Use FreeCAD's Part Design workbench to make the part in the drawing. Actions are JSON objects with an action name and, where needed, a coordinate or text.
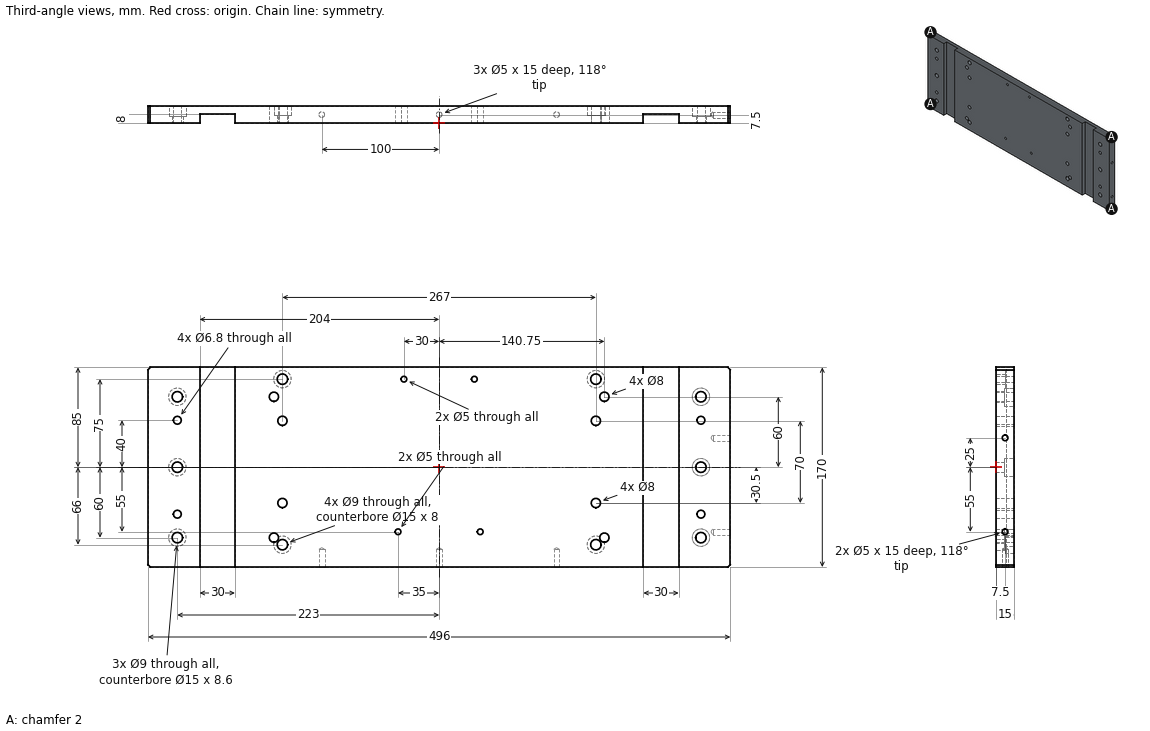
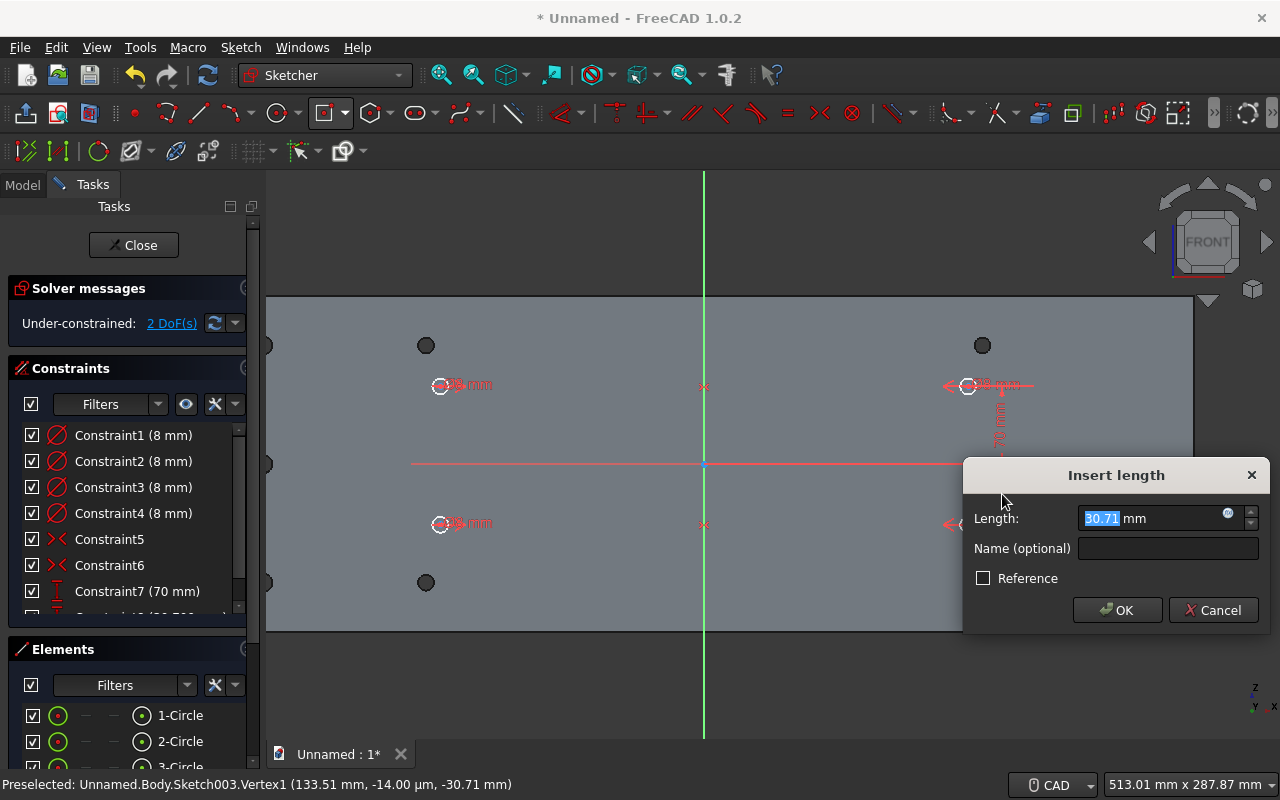
{"action": "type", "text": "30.5"}
{"action": "key", "text": "Return"}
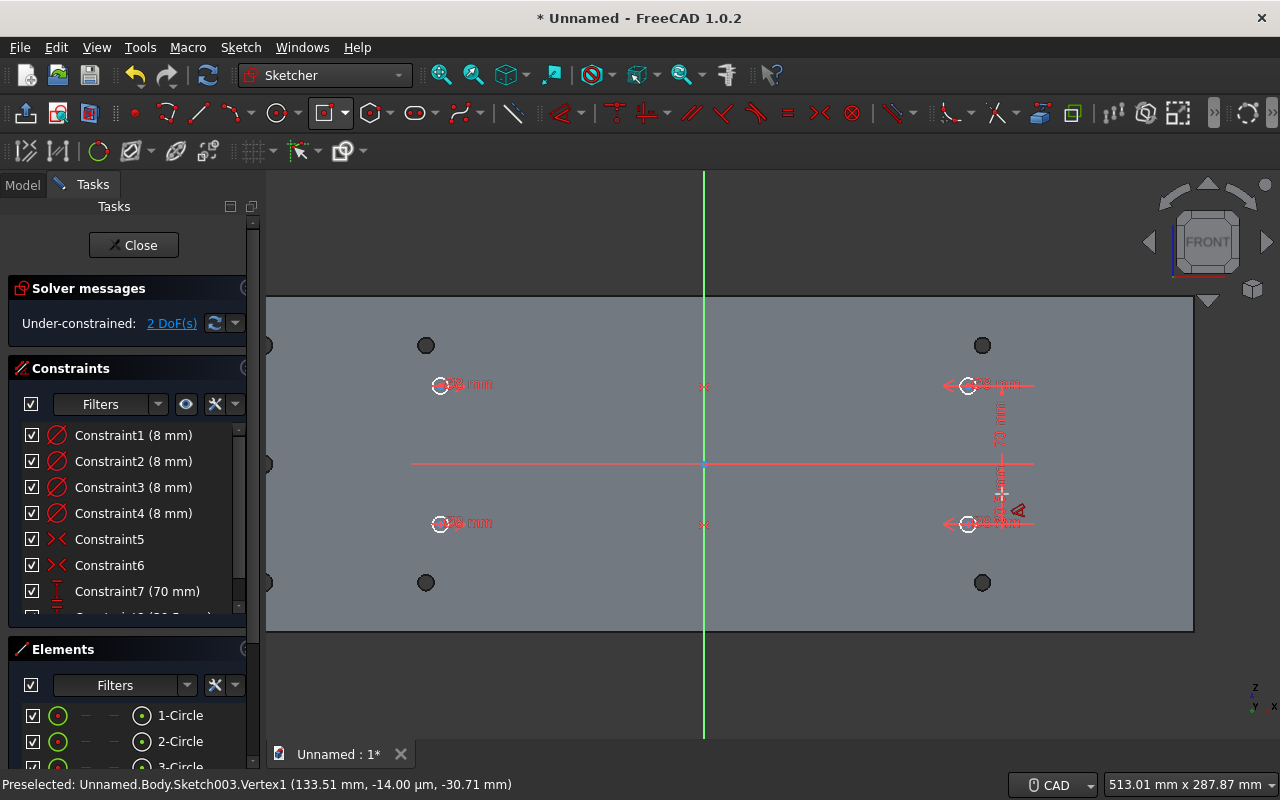
{"action": "left_click", "coordinate": [968, 386]}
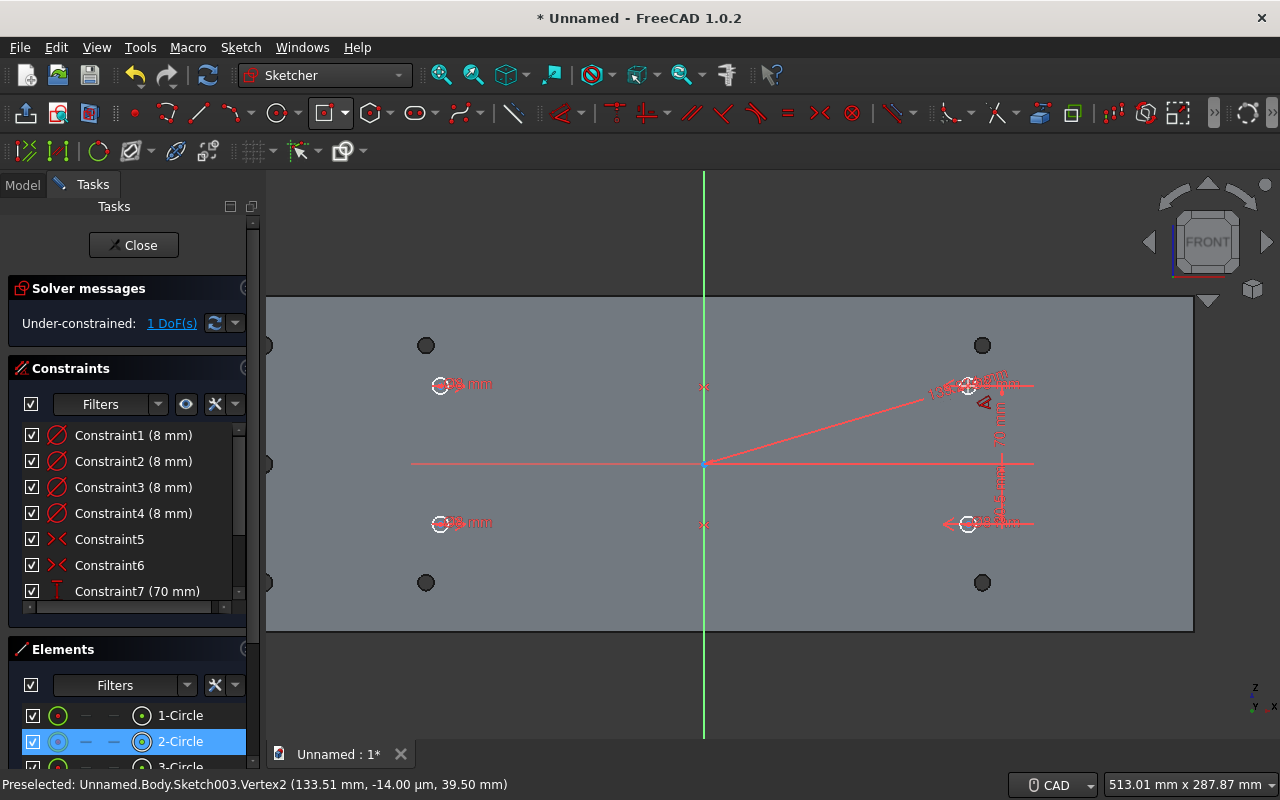
{"action": "left_click", "coordinate": [440, 386]}
{"action": "left_click", "coordinate": [583, 352]}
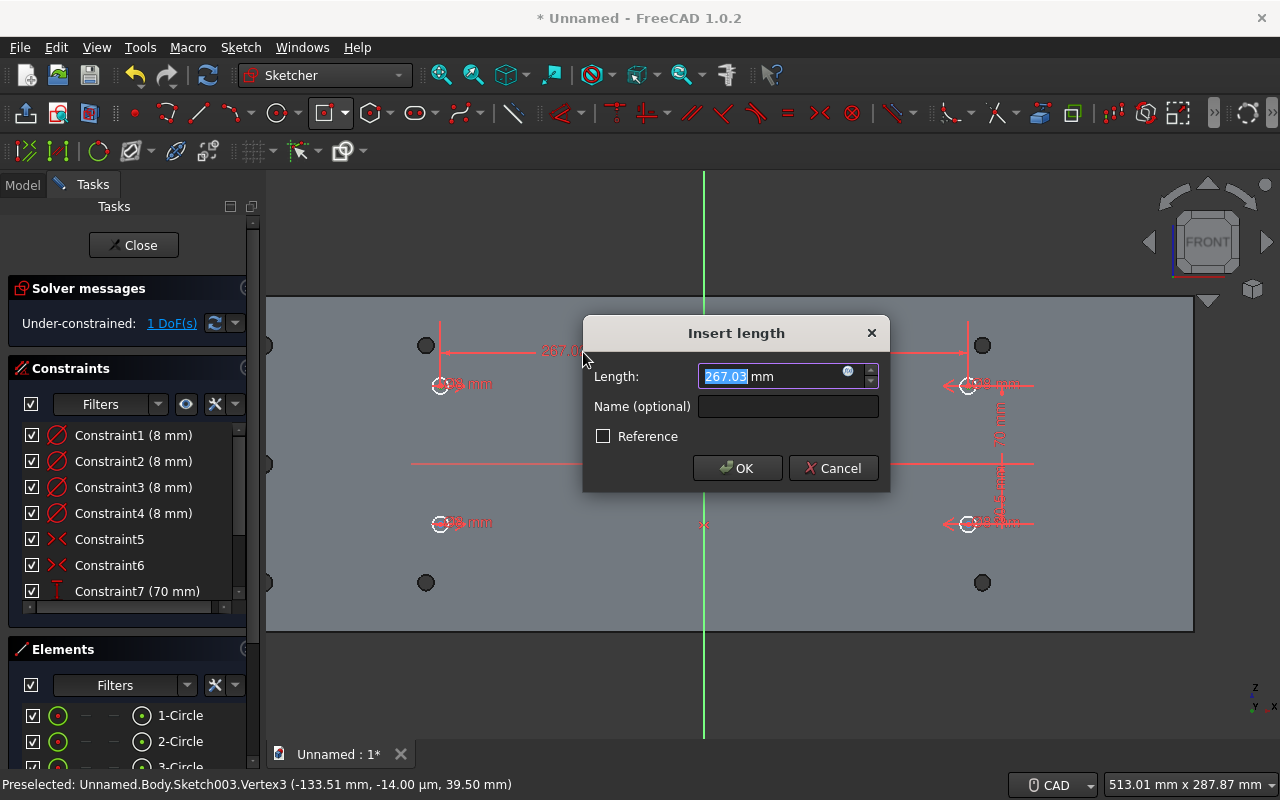
{"action": "type", "text": "267"}
{"action": "key", "text": "Return"}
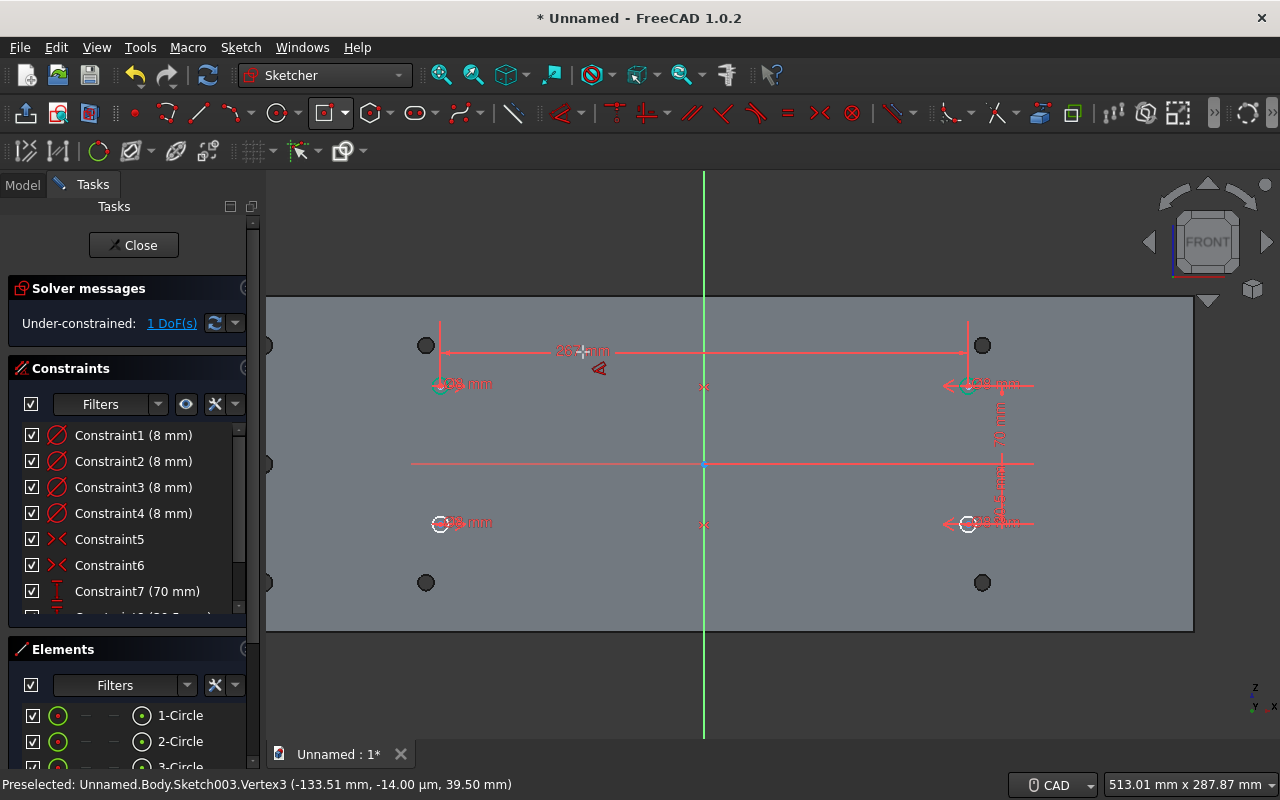
{"action": "left_click", "coordinate": [968, 524]}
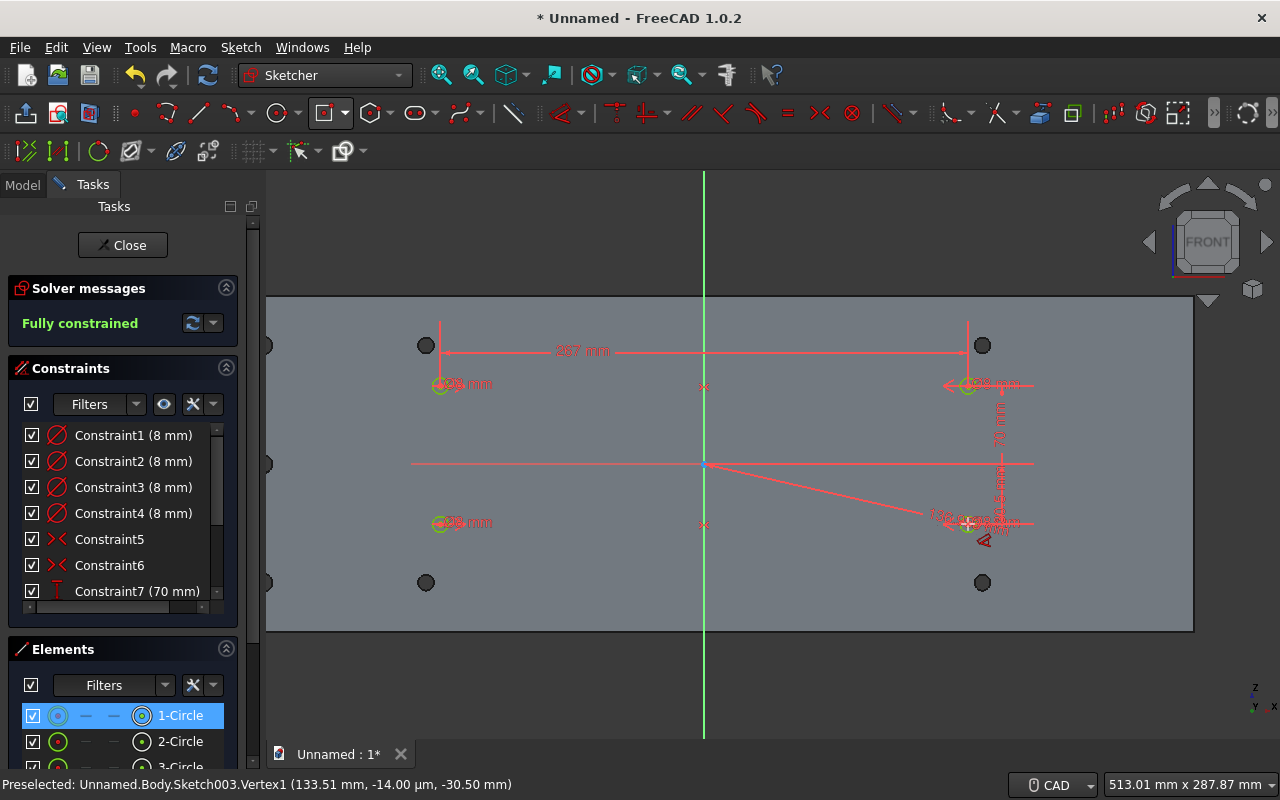
{"action": "left_click", "coordinate": [440, 386]}
{"action": "left_click", "coordinate": [826, 352]}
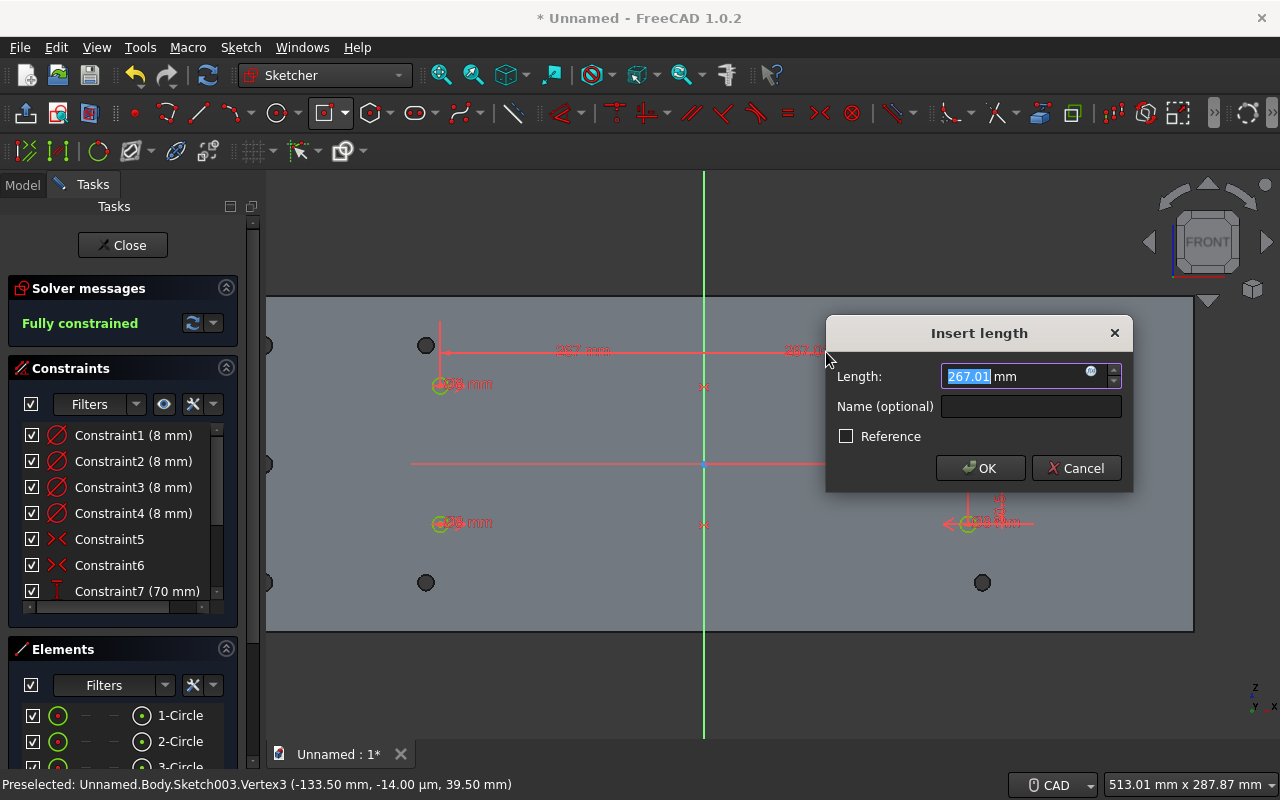
{"action": "type", "text": "267"}
{"action": "key", "text": "Return"}
{"action": "key", "text": "Escape"}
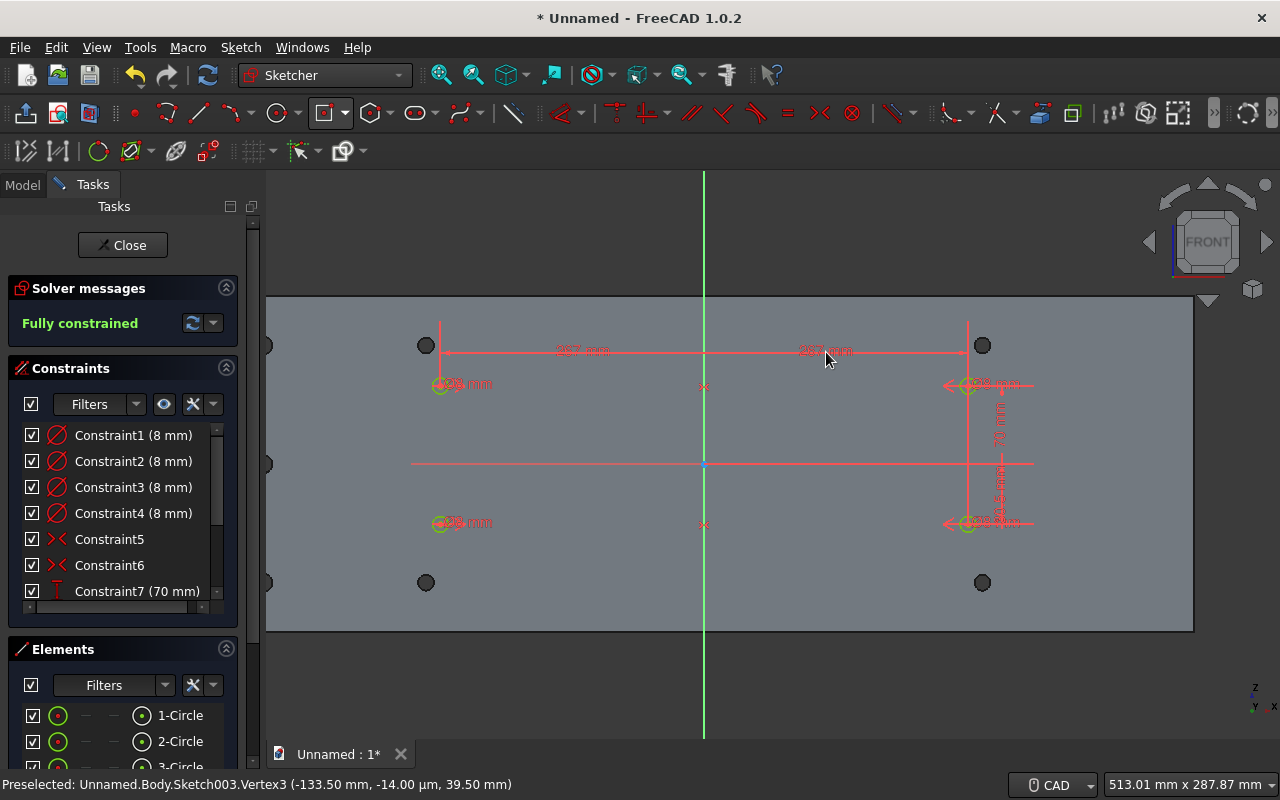
{"action": "left_click", "coordinate": [123, 245]}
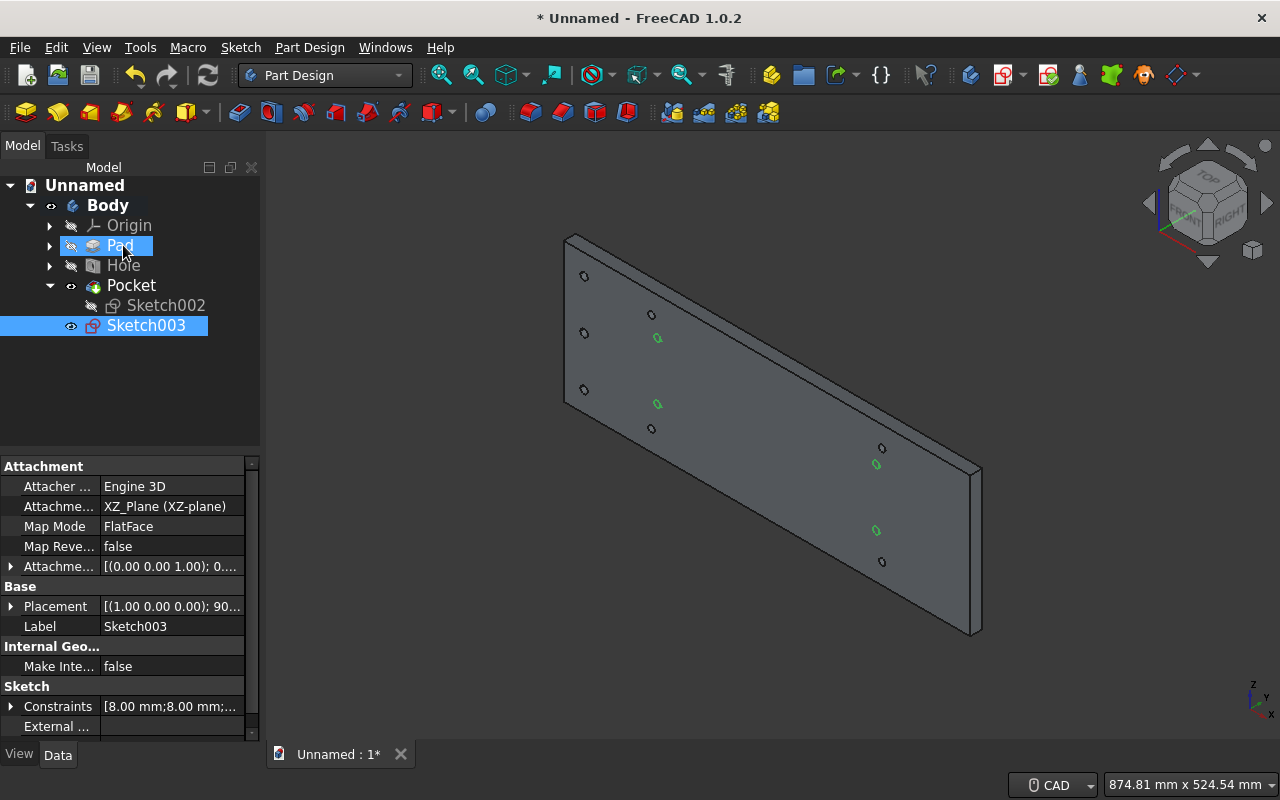
{"action": "left_click", "coordinate": [240, 112]}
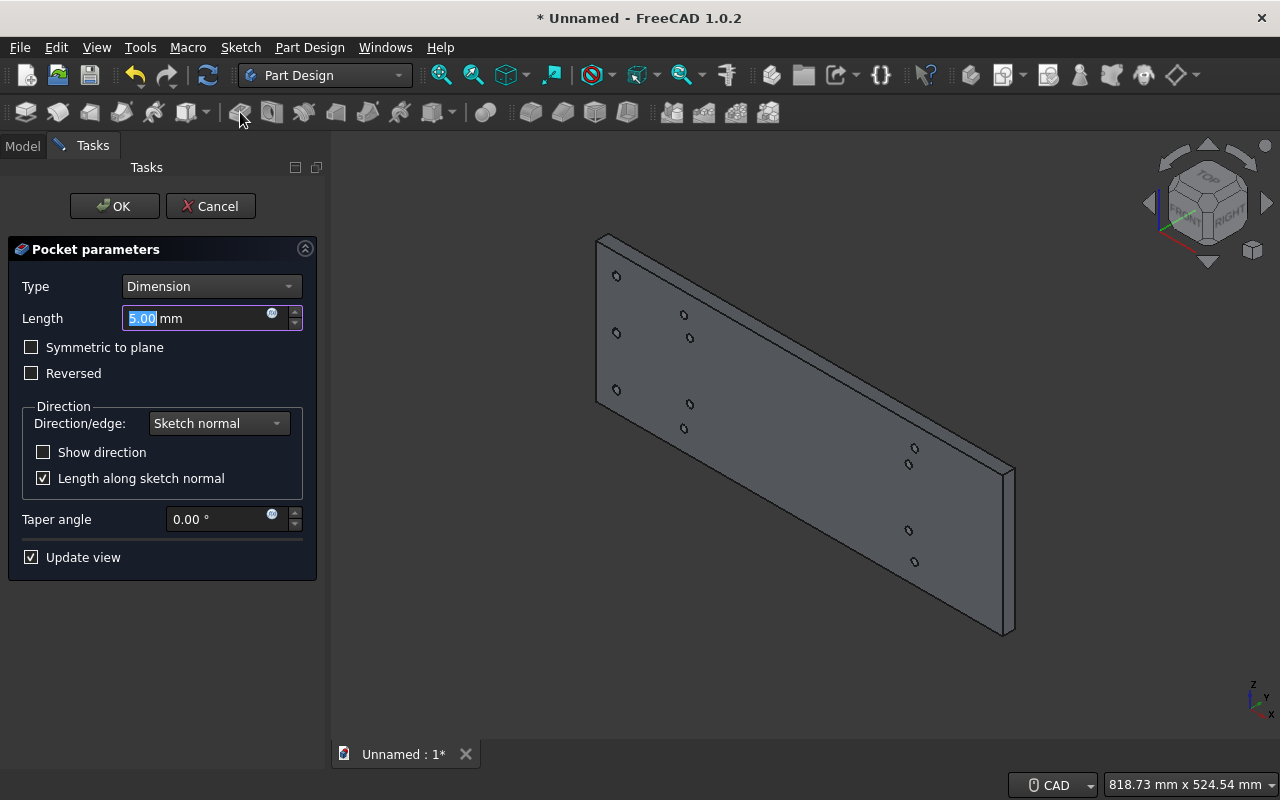
{"action": "left_click", "coordinate": [212, 286]}